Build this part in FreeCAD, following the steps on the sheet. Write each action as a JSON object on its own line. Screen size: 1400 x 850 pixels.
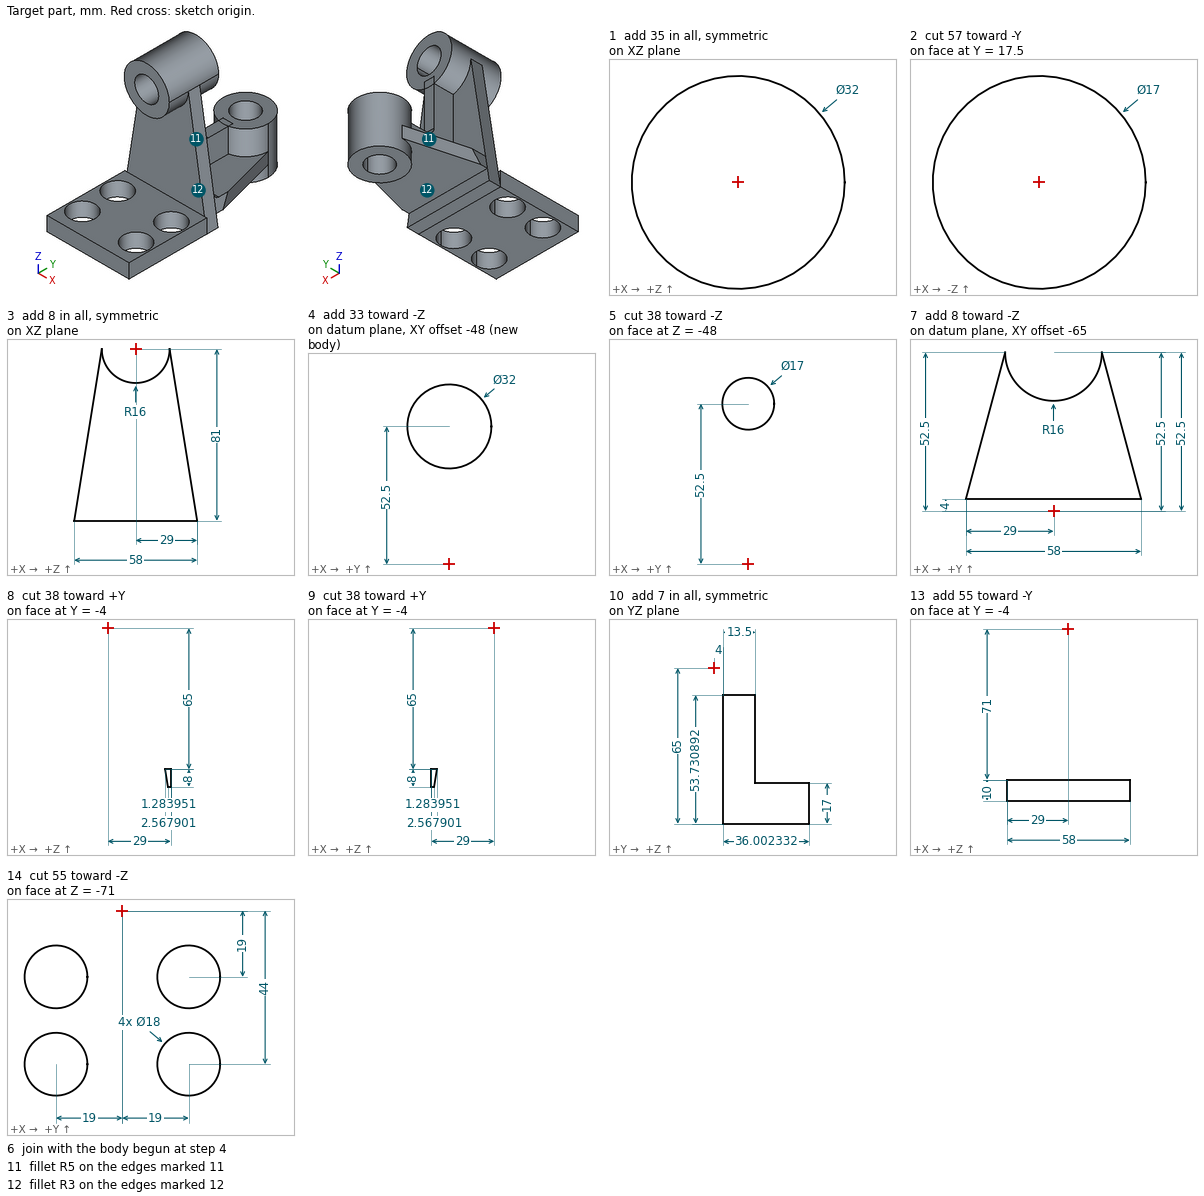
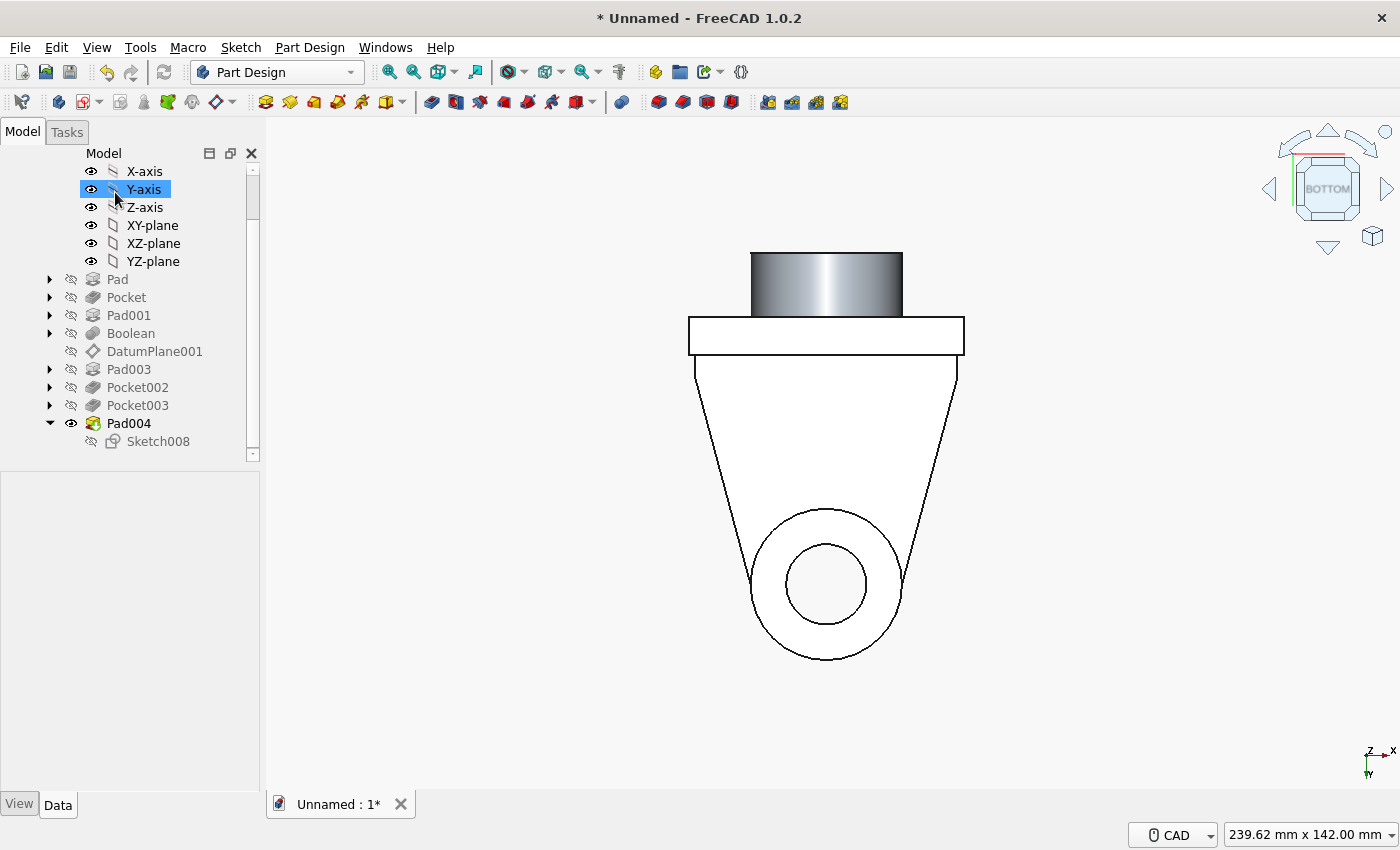
{"action": "key", "text": "4"}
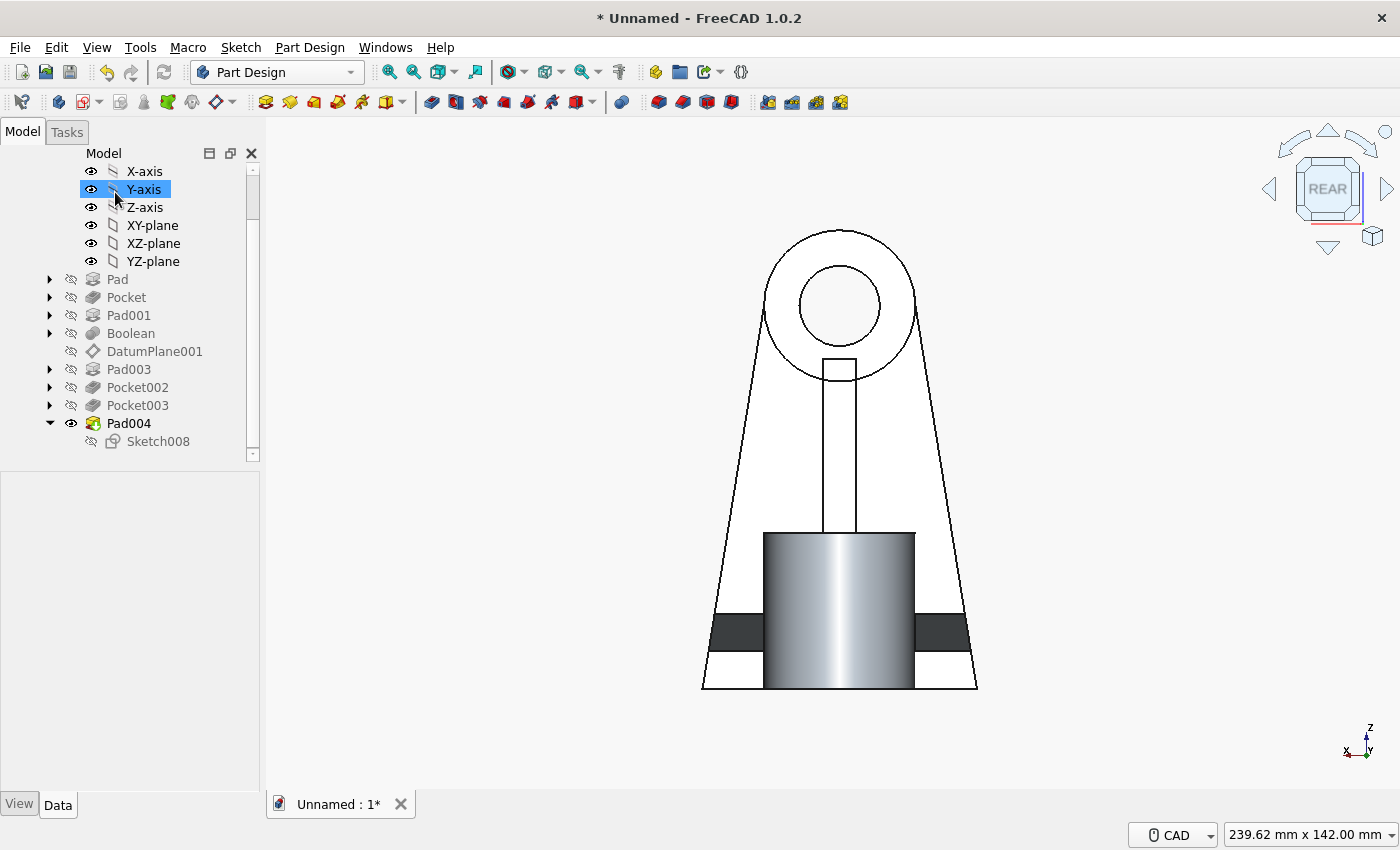
{"action": "key", "text": "6"}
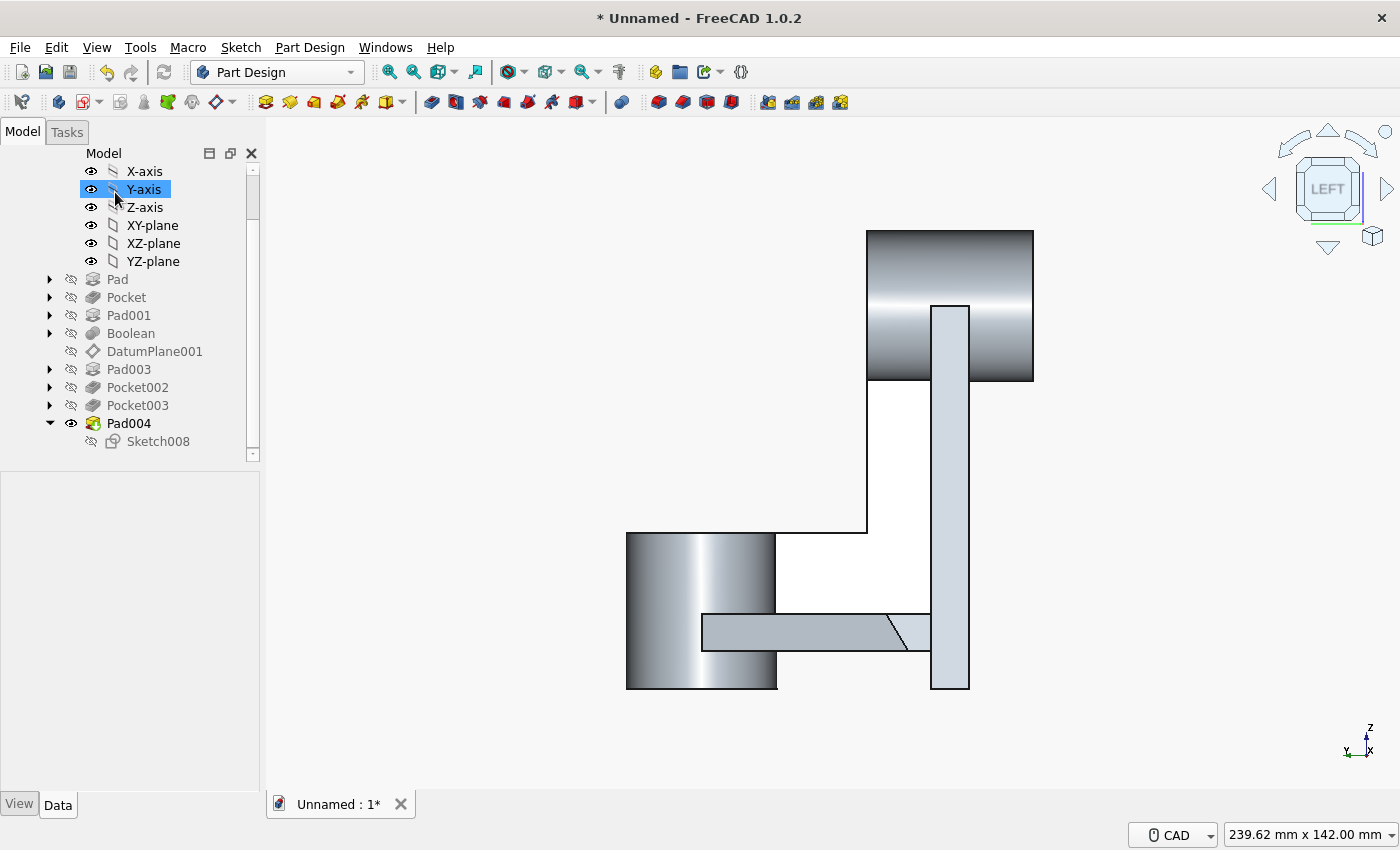
{"action": "key", "text": "v 3"}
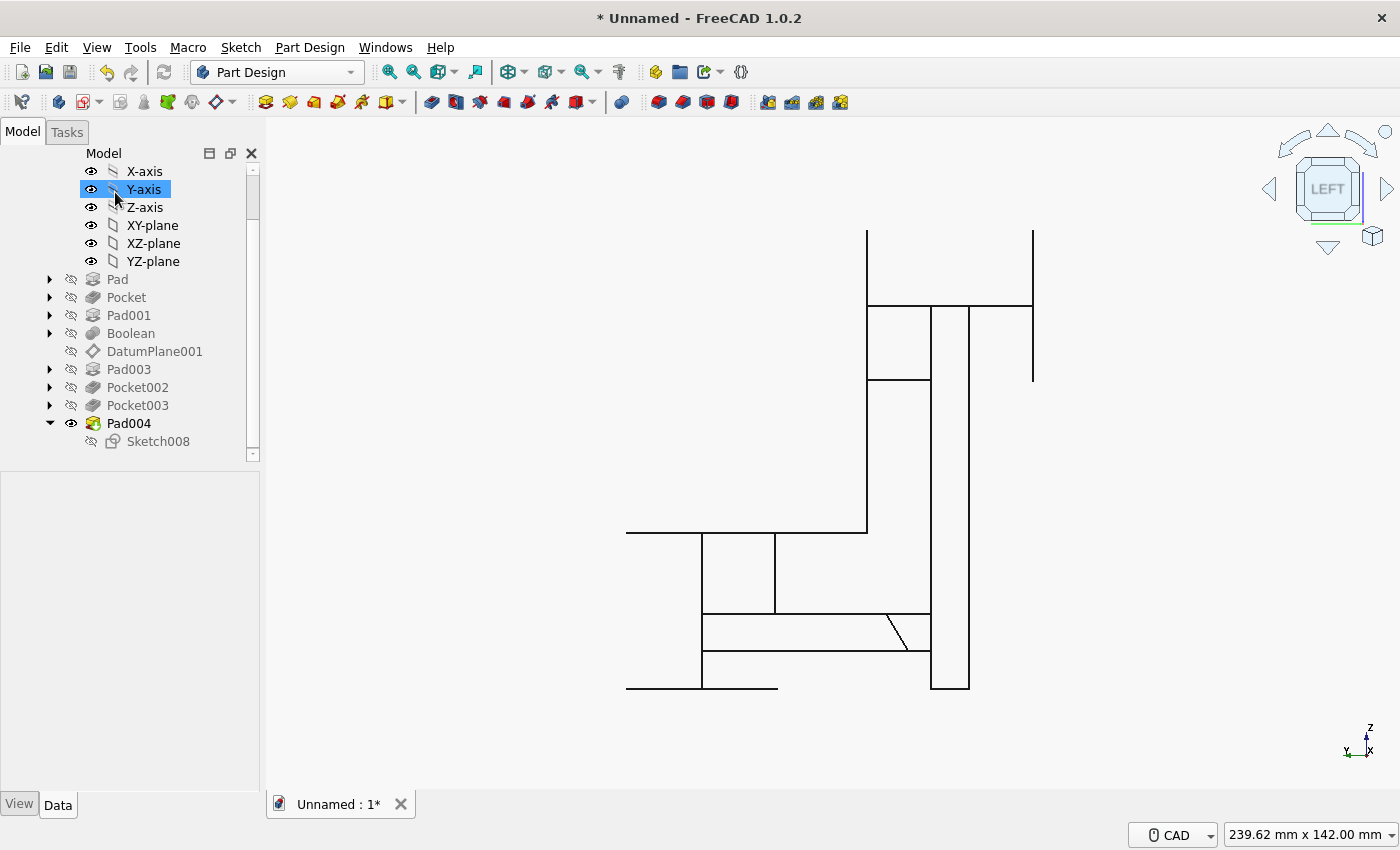
{"action": "key", "text": "0"}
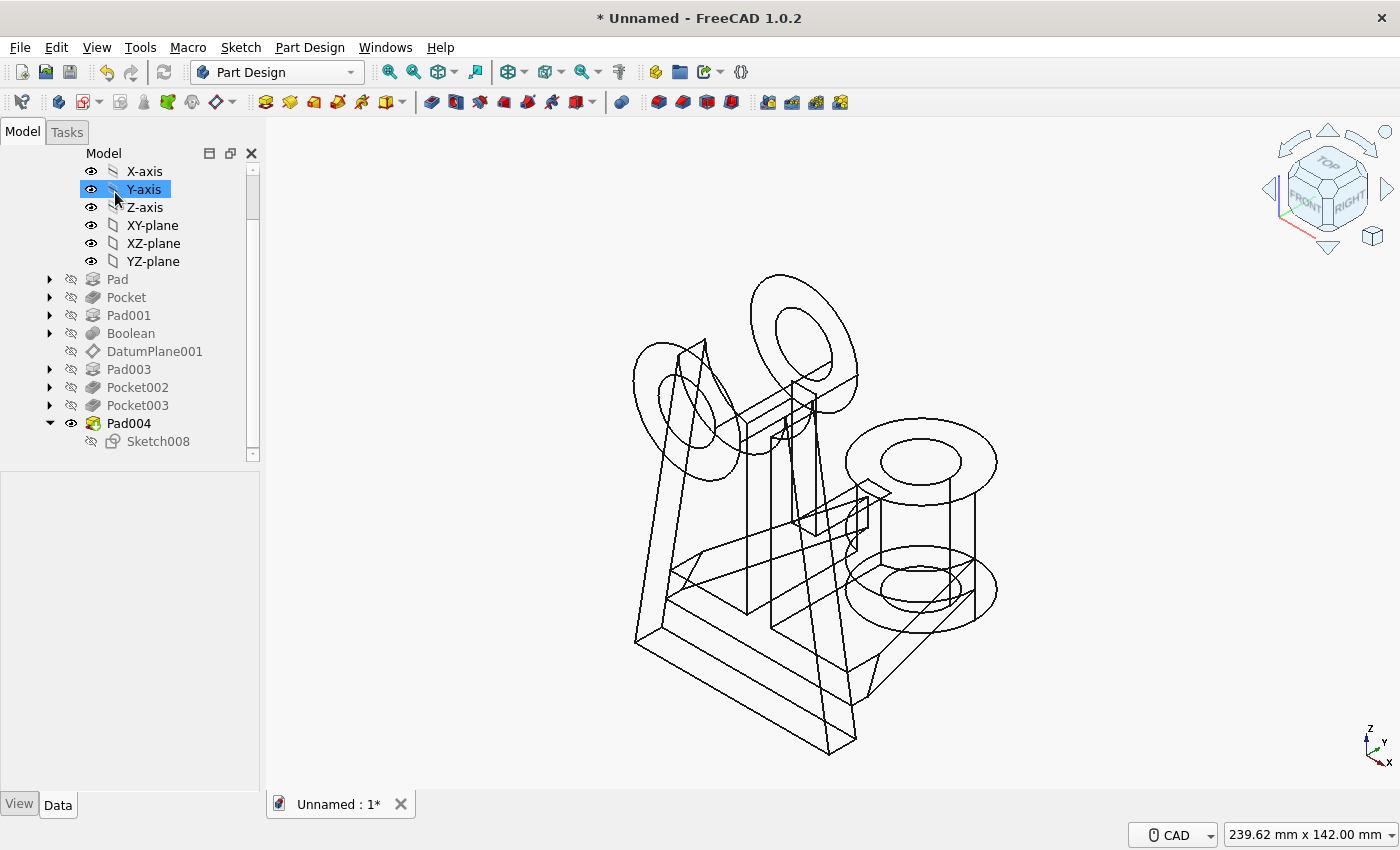
{"action": "left_click", "coordinate": [809, 531]}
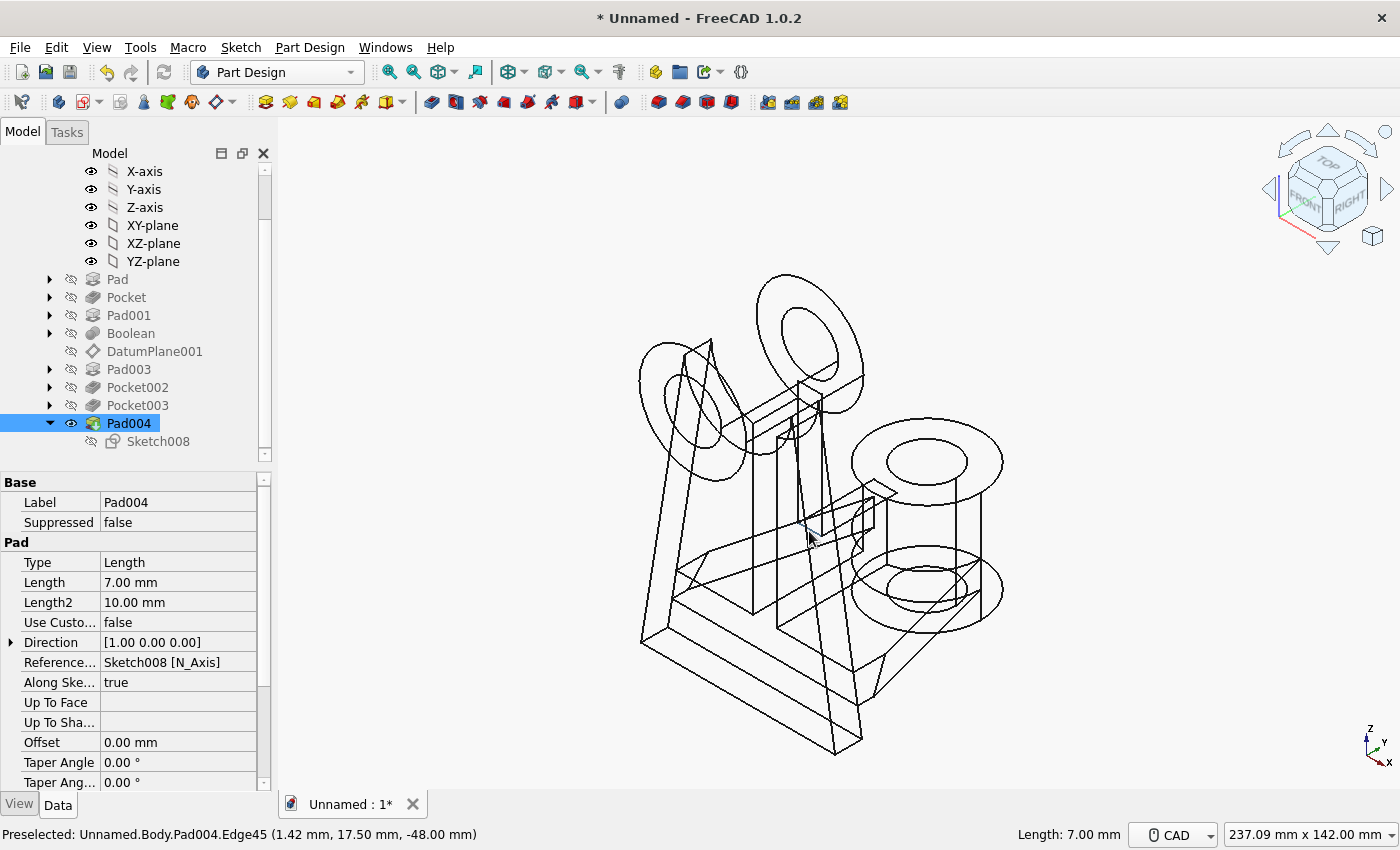
{"action": "key", "text": "v 1"}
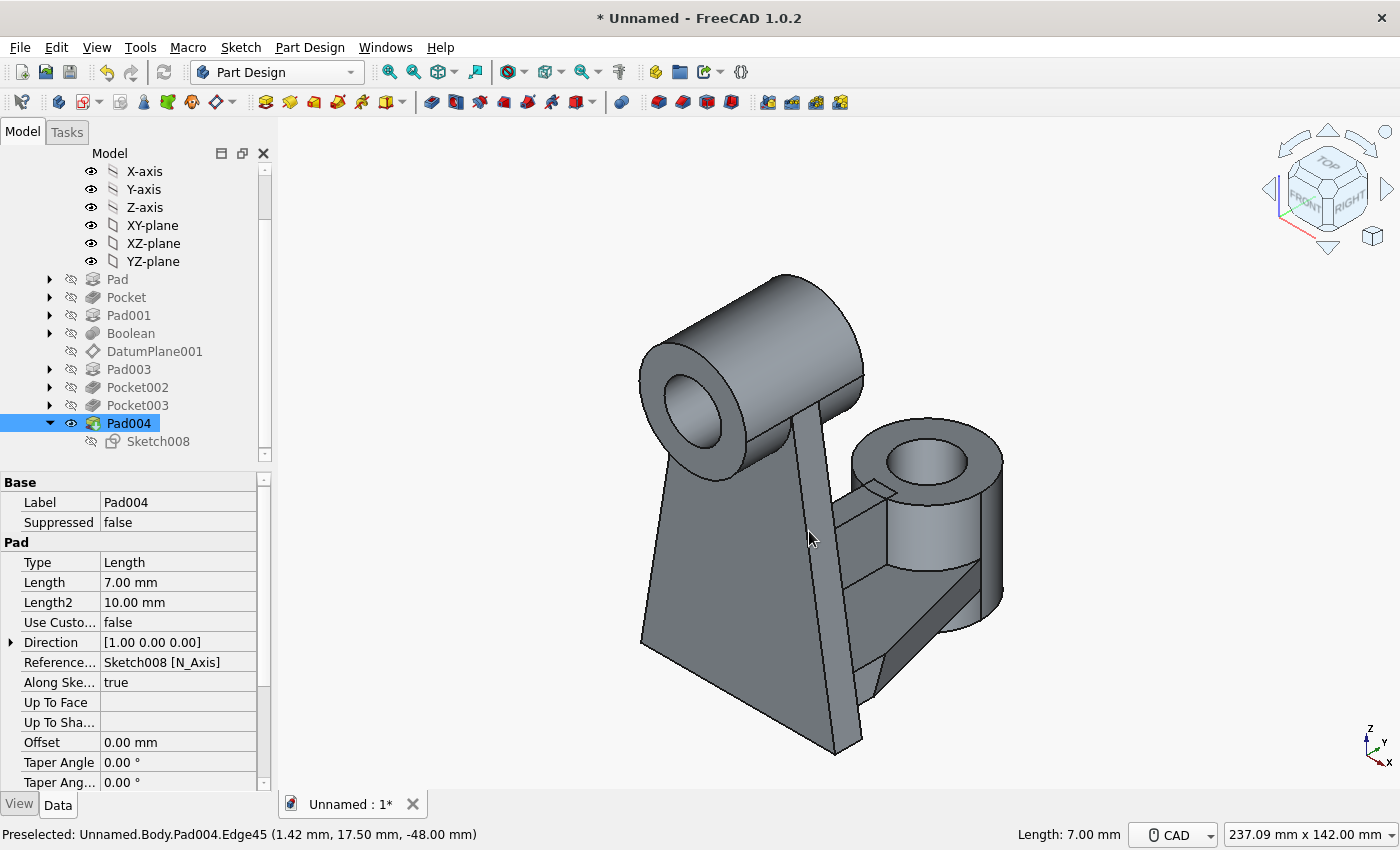
{"action": "left_click", "coordinate": [660, 102]}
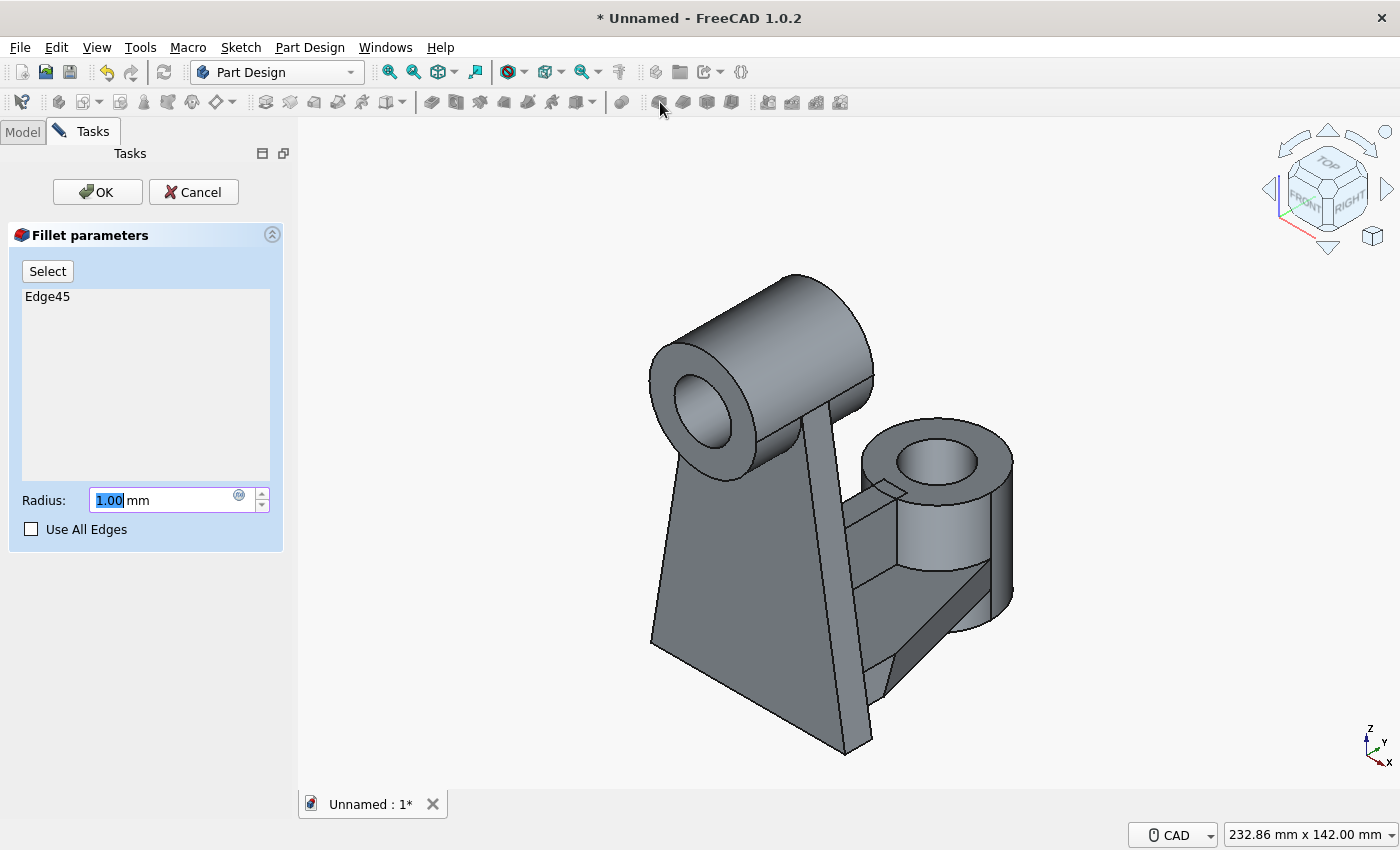
{"action": "type", "text": "5"}
{"action": "key", "text": "Tab"}